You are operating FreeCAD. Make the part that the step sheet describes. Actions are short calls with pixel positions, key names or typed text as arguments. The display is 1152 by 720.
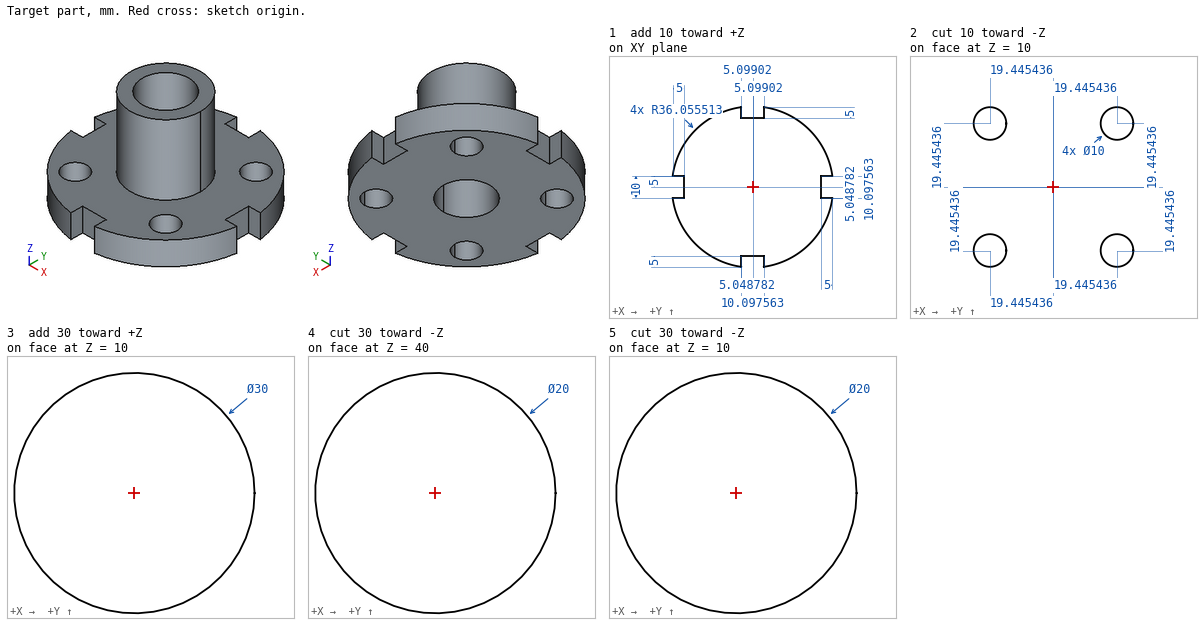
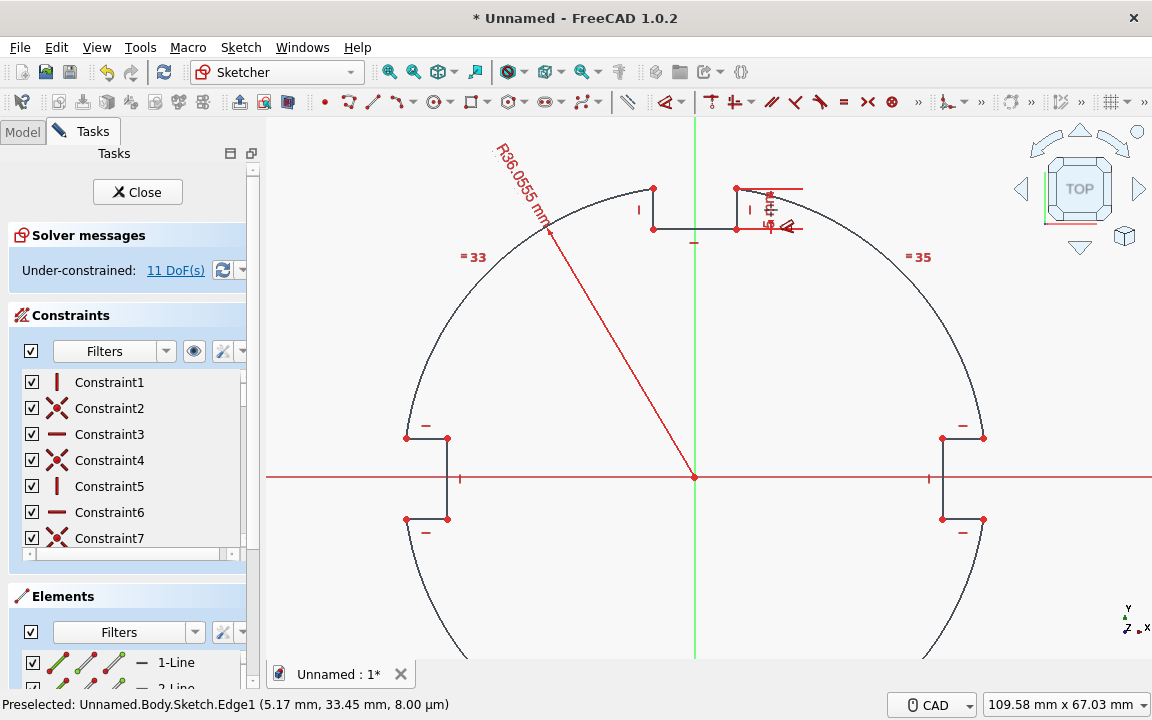
click(418, 439)
click(427, 405)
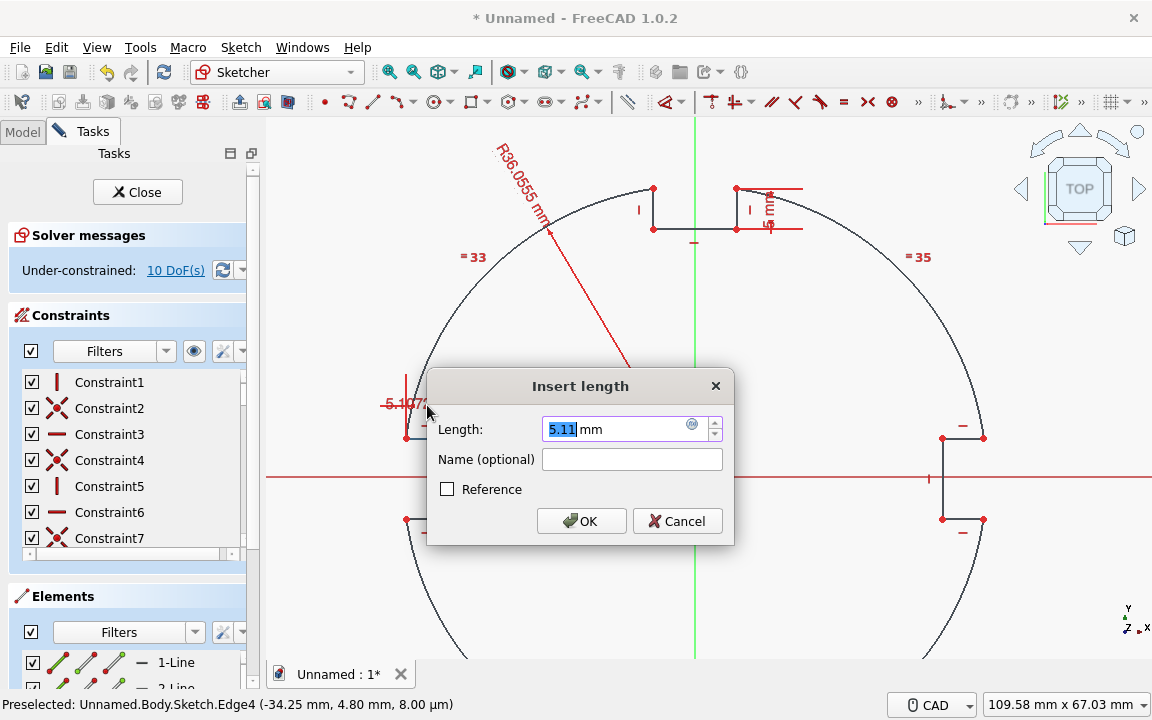
text(5)
key(Return)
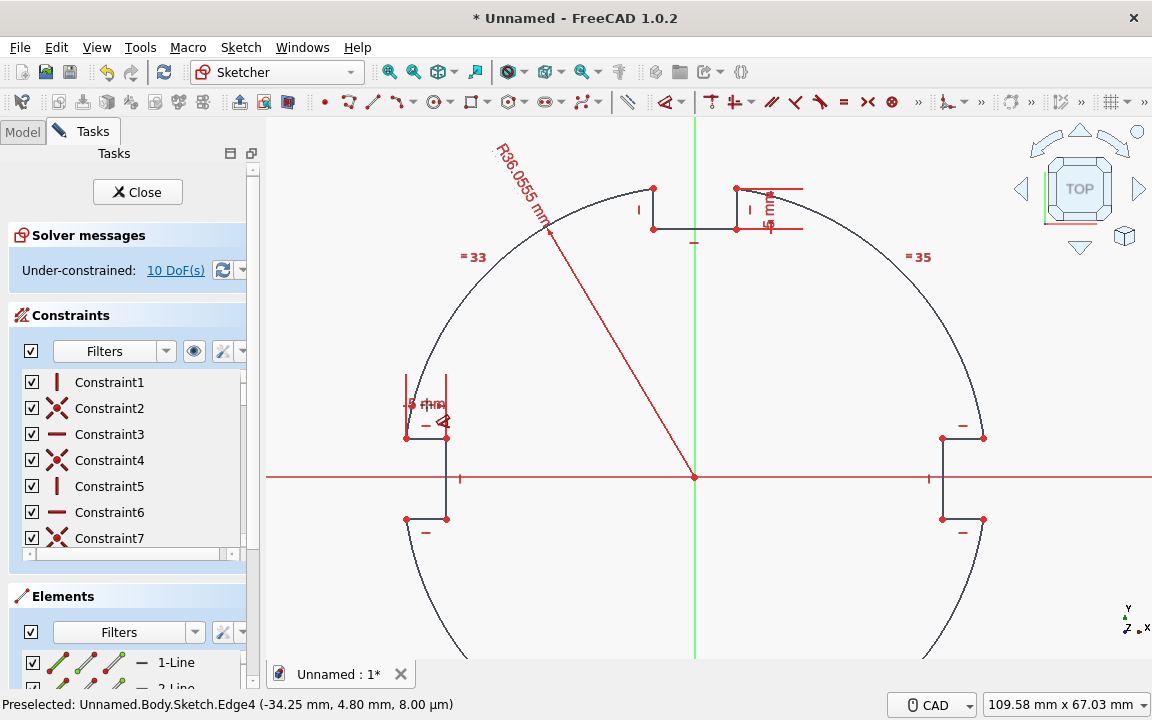
scroll(574, 279, down, 3)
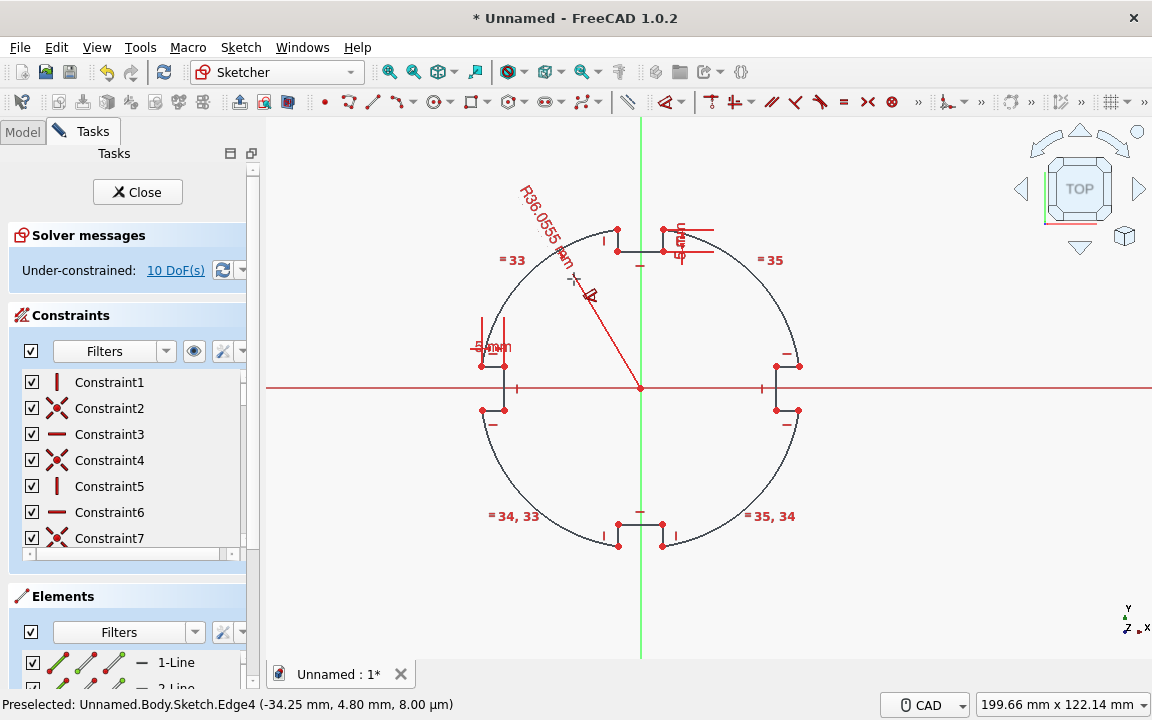
scroll(618, 540, up, 4)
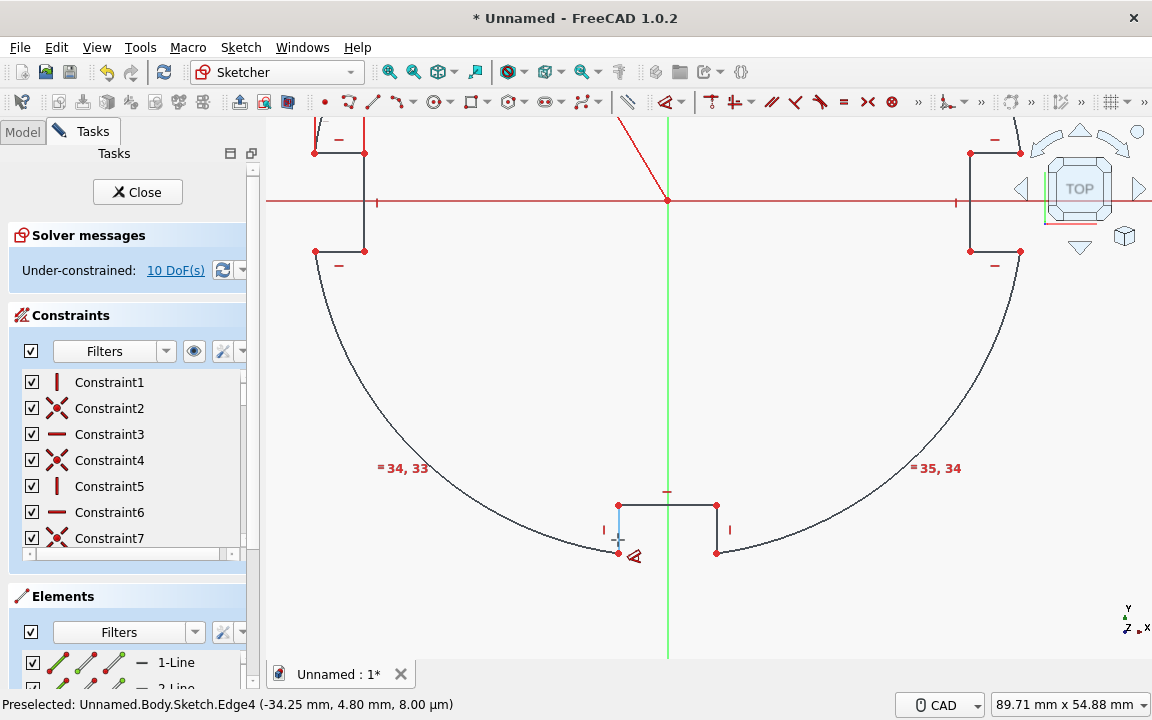
click(619, 539)
click(585, 529)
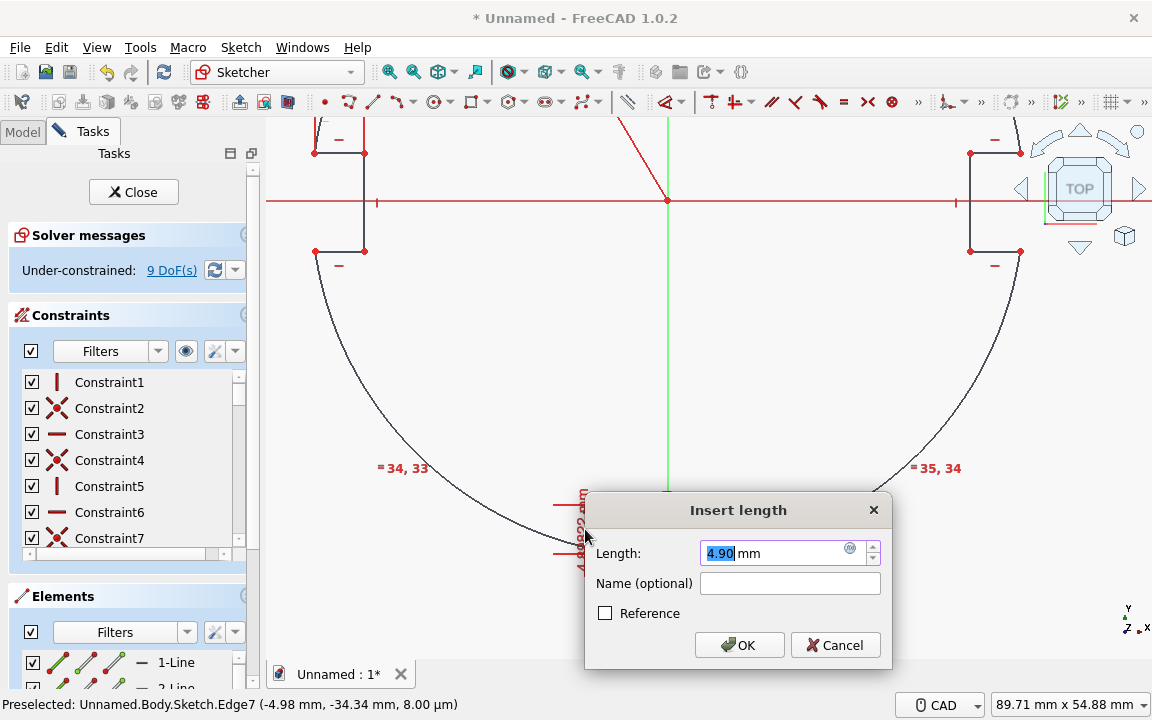
text(5)
key(Return)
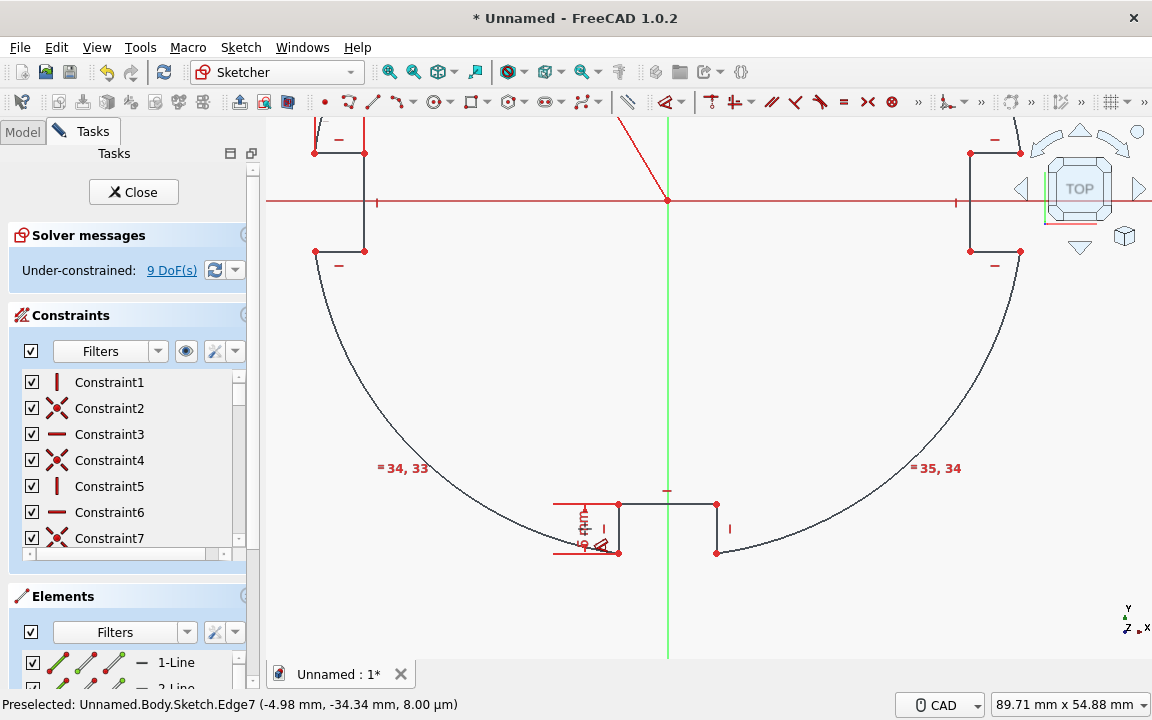
click(985, 252)
click(979, 286)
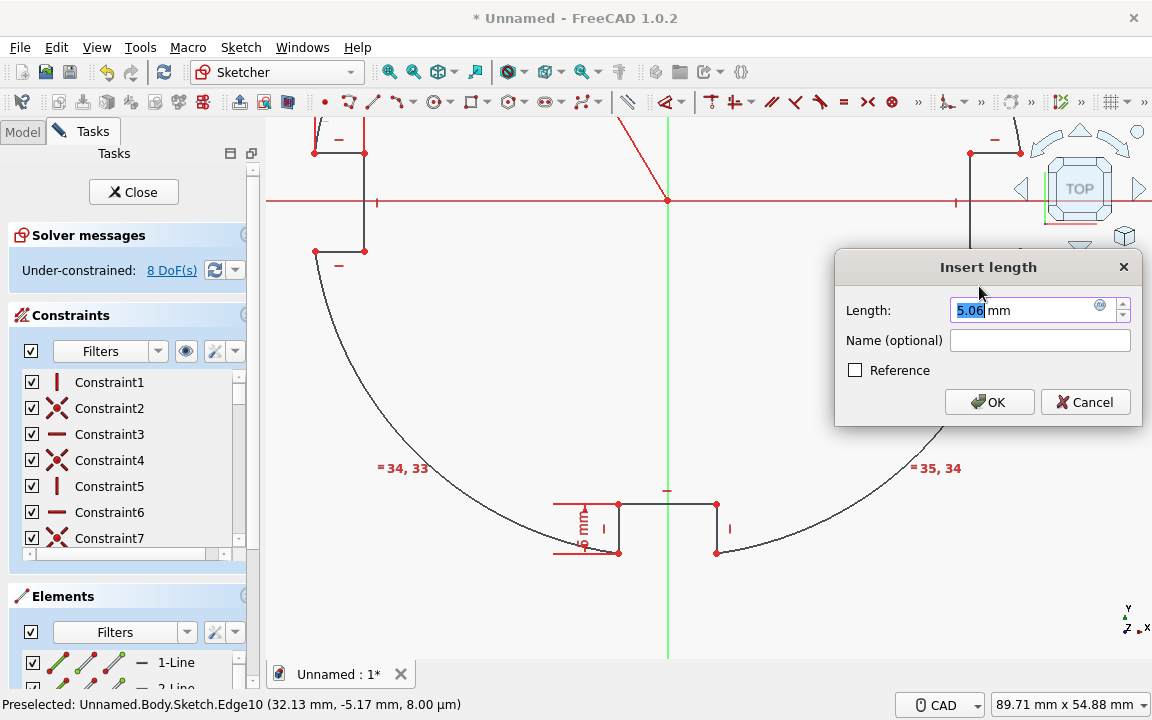
text(5)
key(Return)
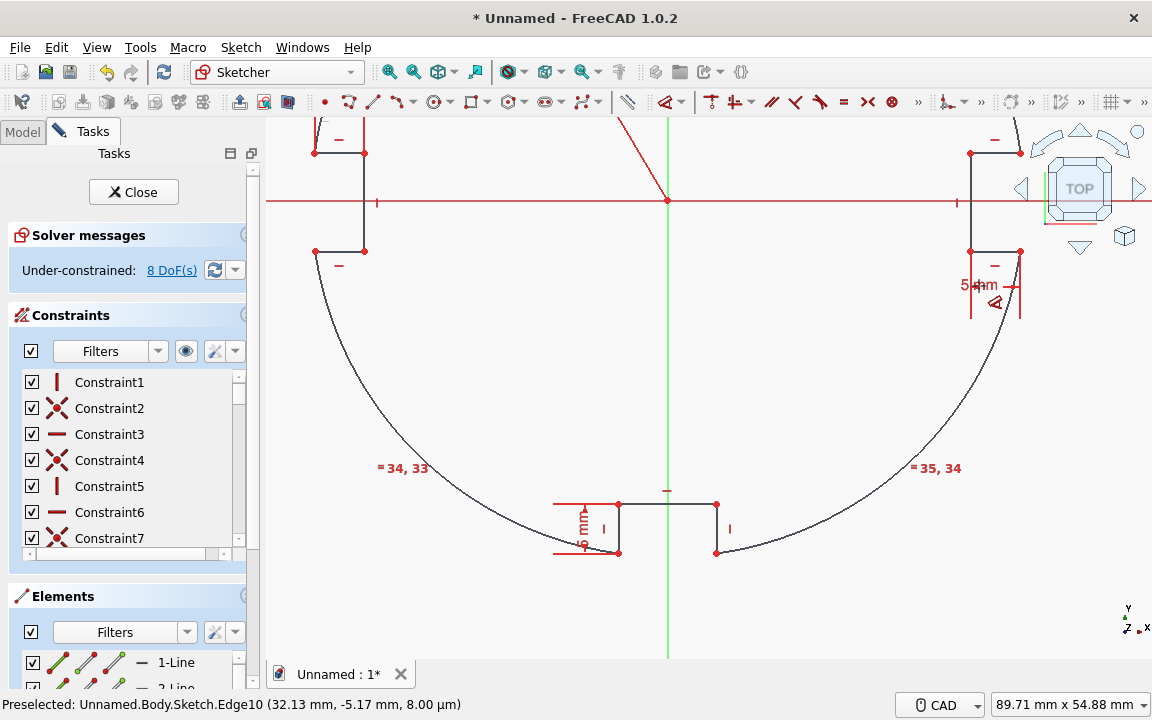
click(364, 183)
click(330, 180)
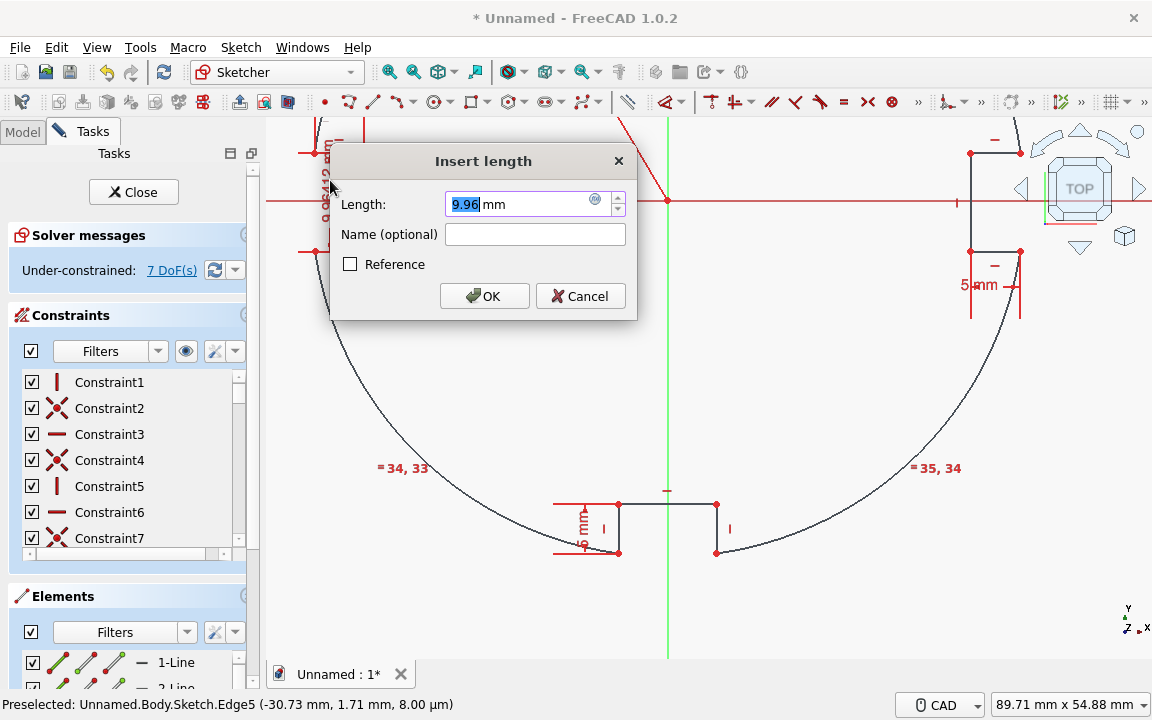
text(10)
key(Return)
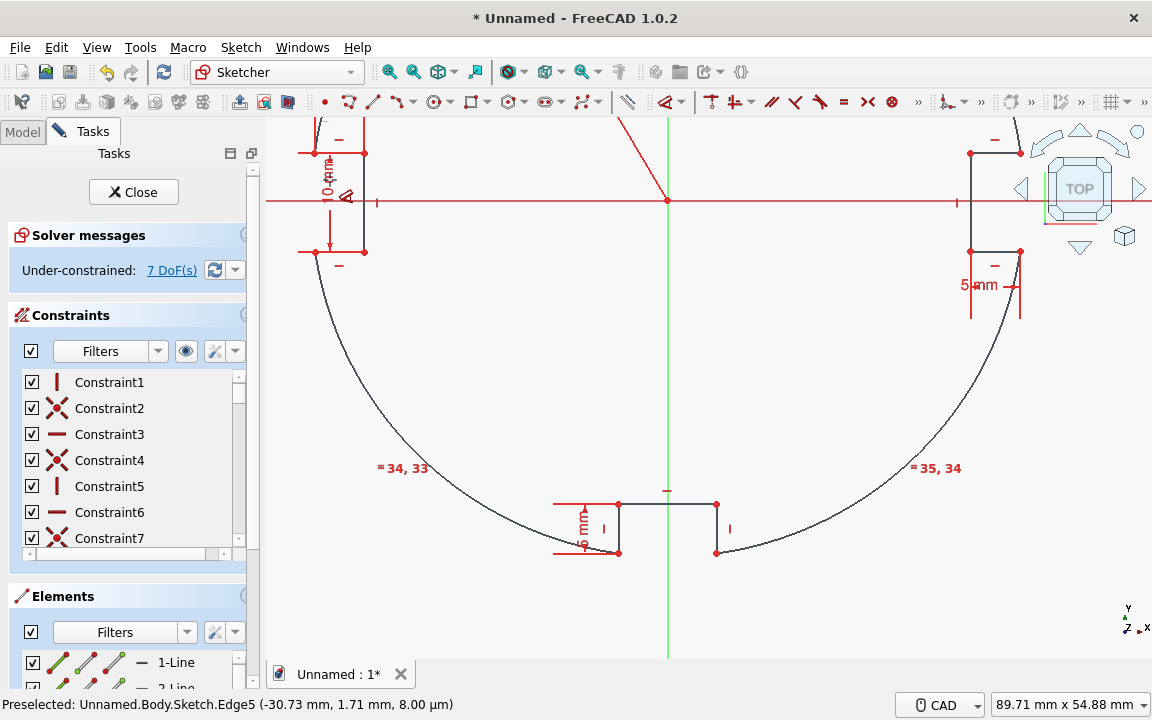
click(315, 153)
click(702, 177)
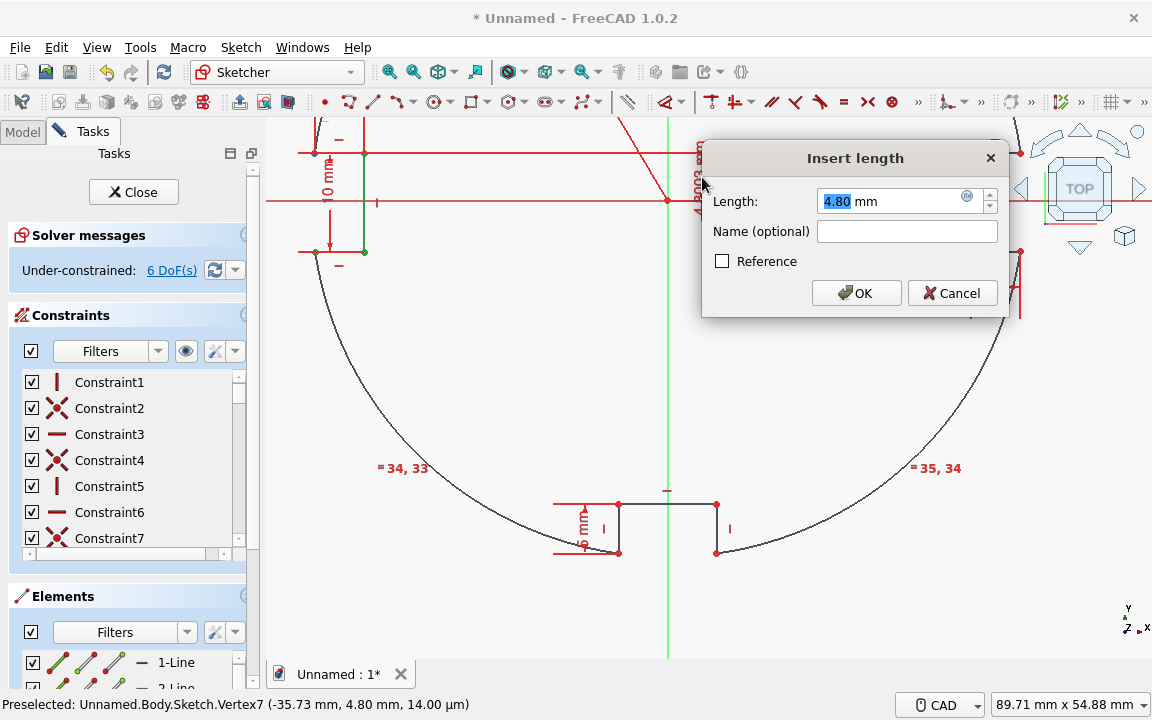
text(5)
key(Return)